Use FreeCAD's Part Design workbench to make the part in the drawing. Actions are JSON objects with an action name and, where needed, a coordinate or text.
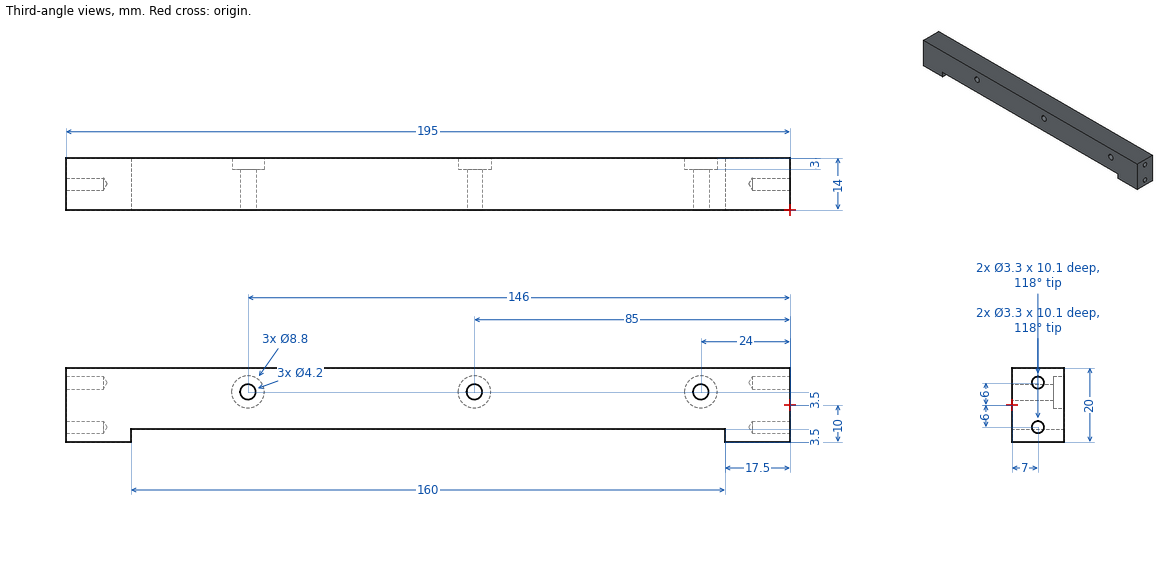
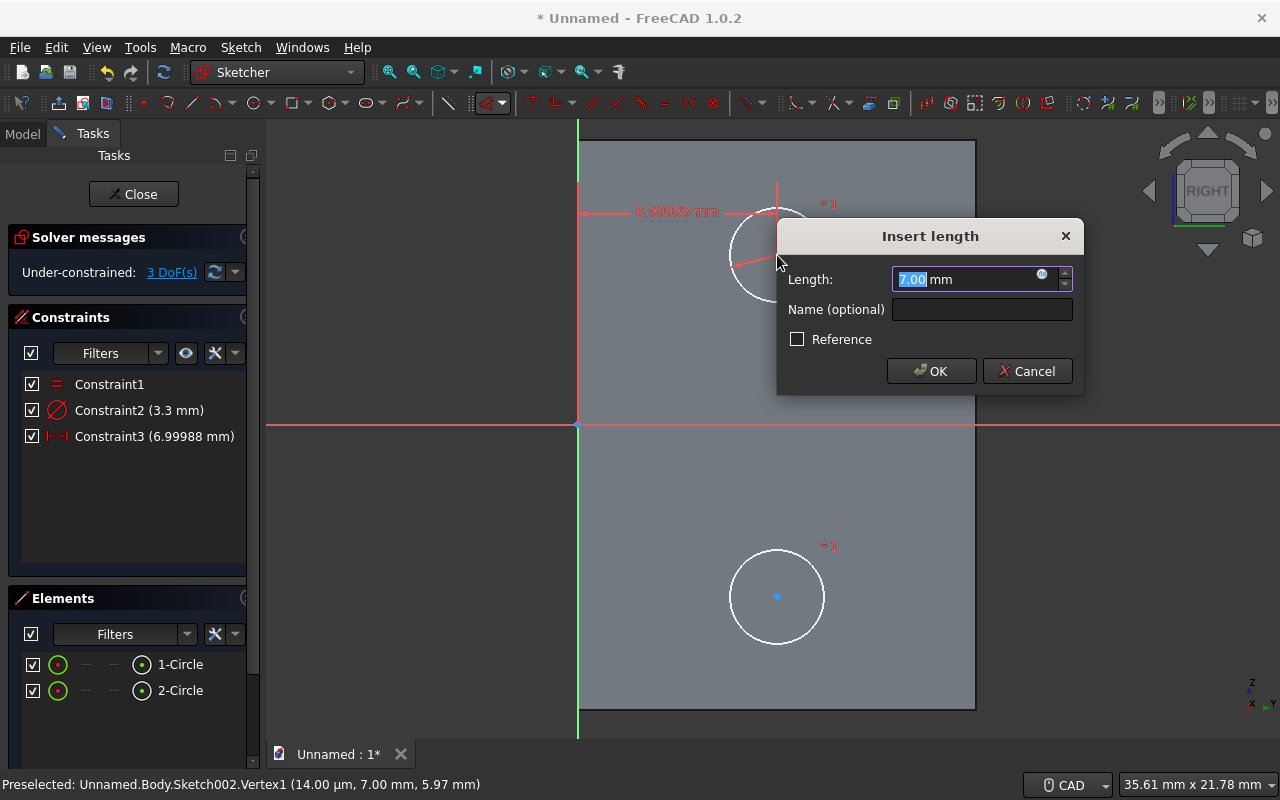
{"action": "type", "text": "7"}
{"action": "key", "text": "Return"}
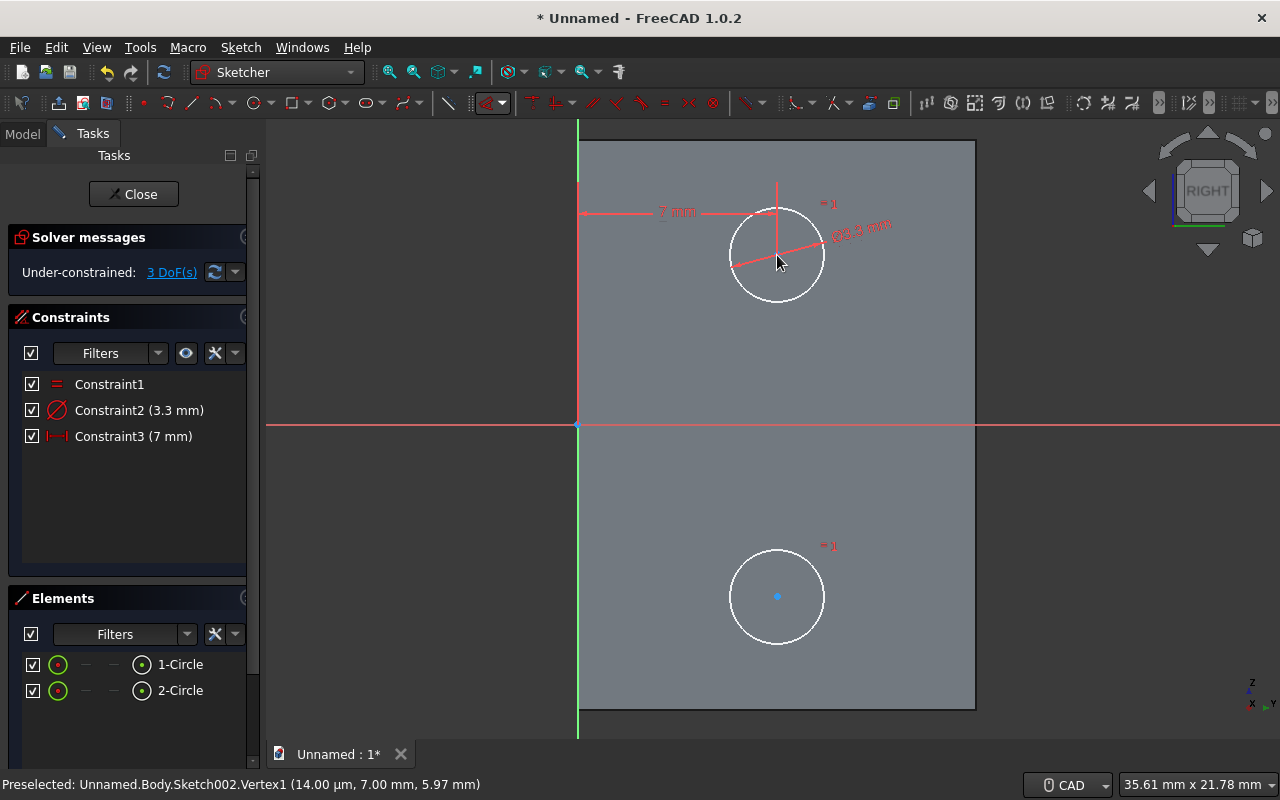
{"action": "left_click", "coordinate": [777, 255]}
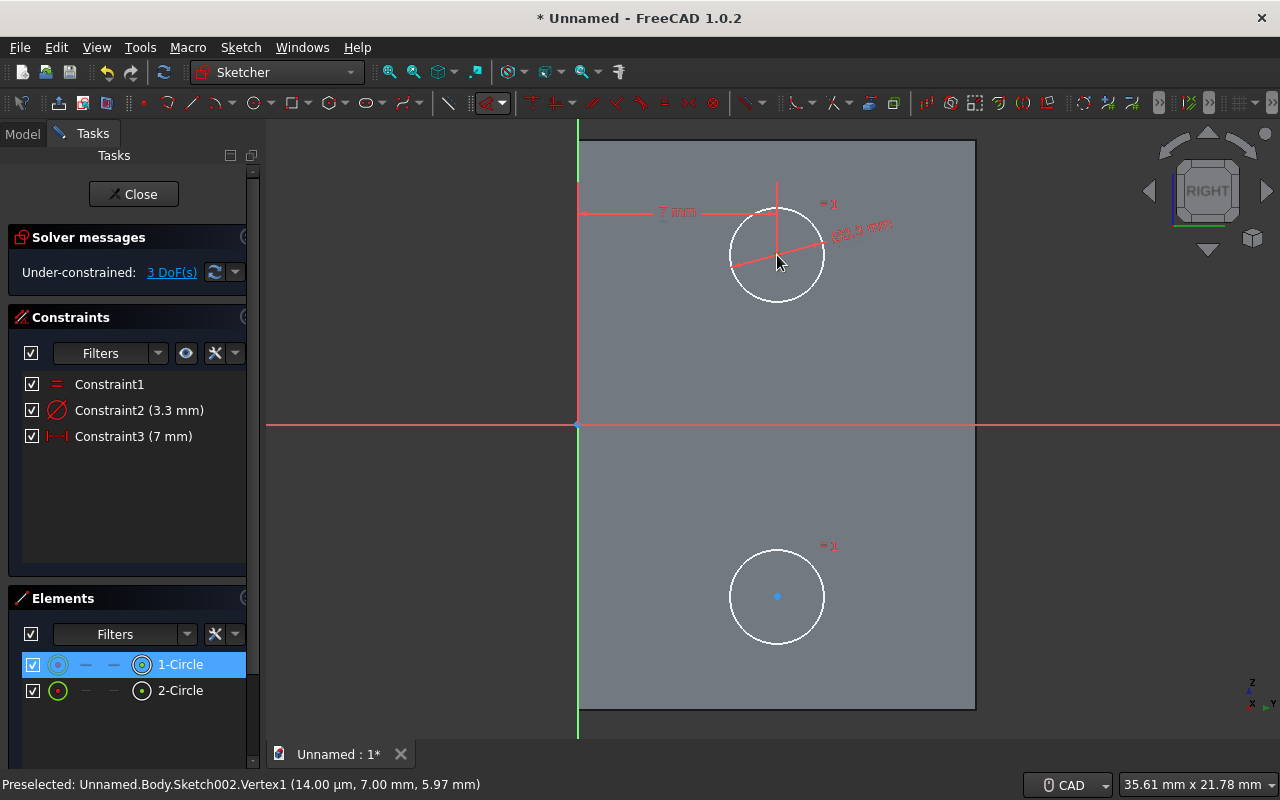
{"action": "key", "text": "i"}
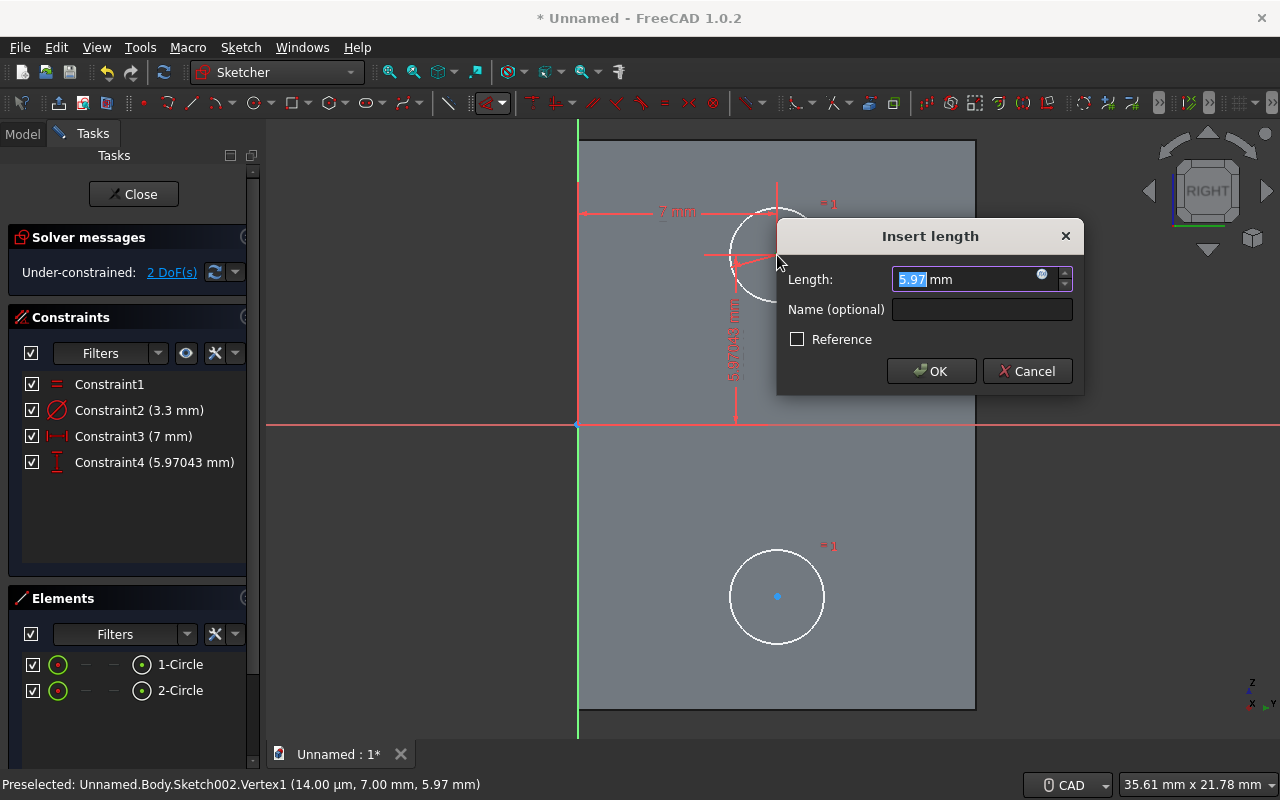
{"action": "type", "text": "6"}
{"action": "key", "text": "Return"}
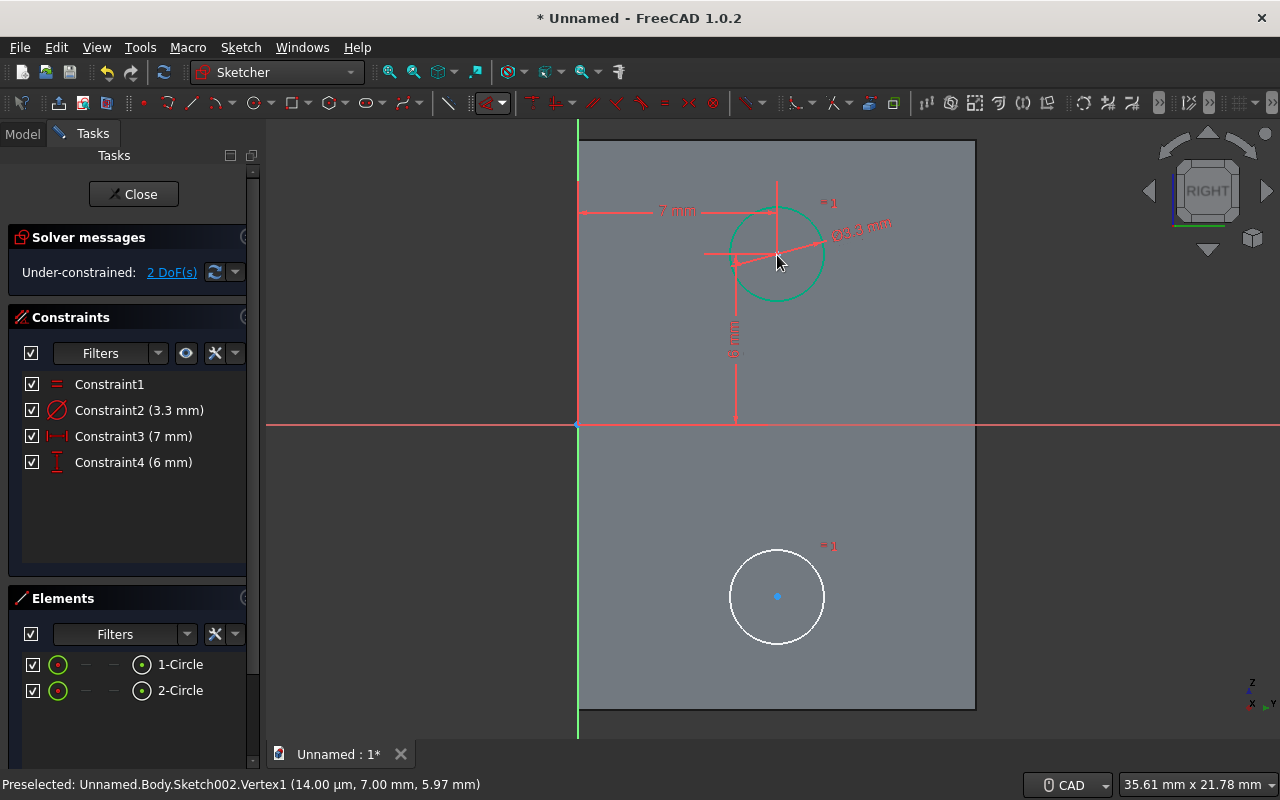
{"action": "left_click", "coordinate": [777, 597]}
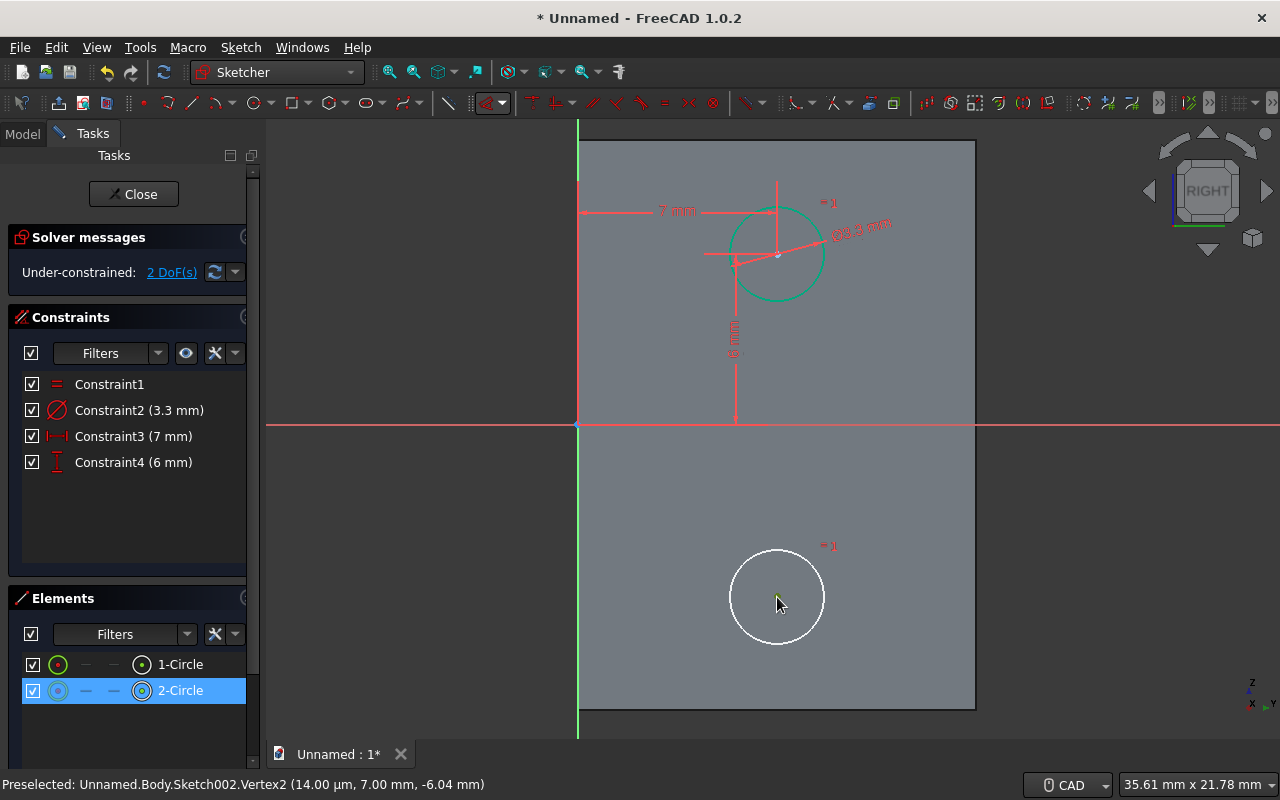
{"action": "key", "text": "l"}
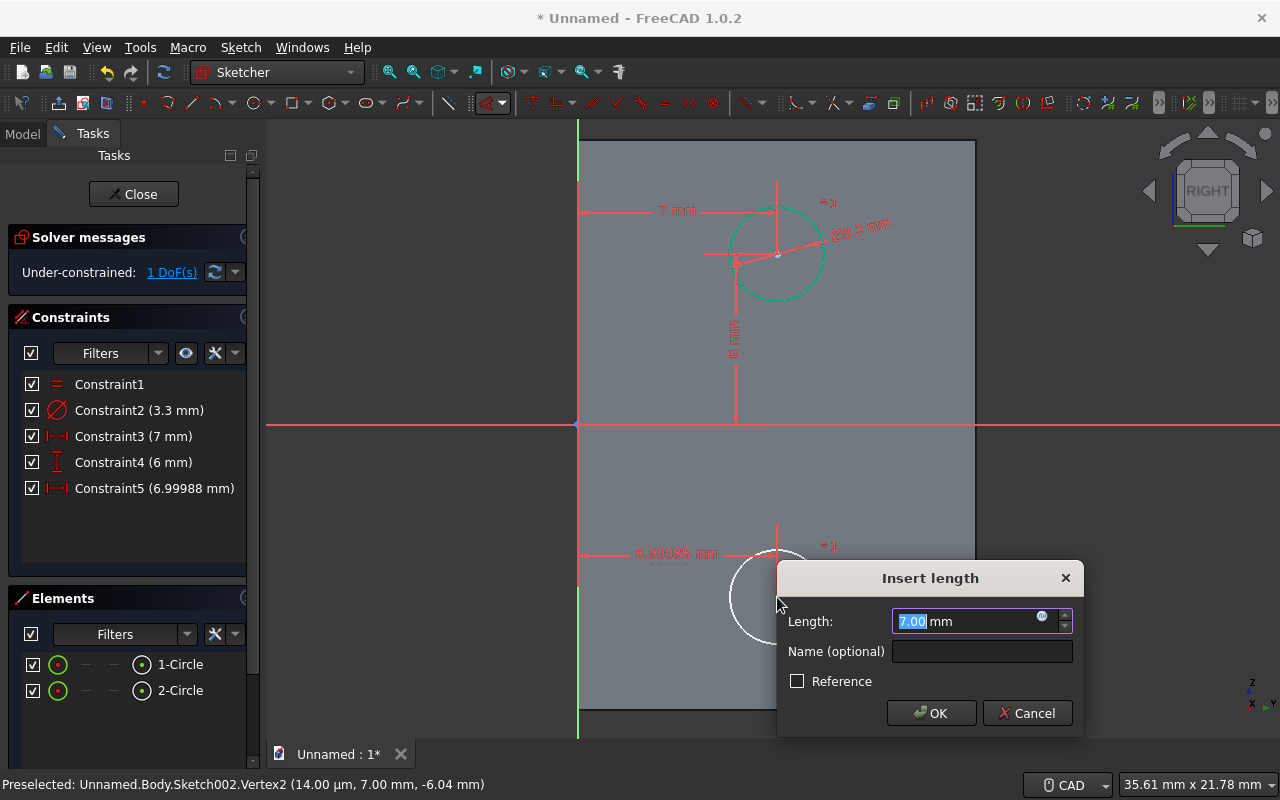
{"action": "type", "text": "7"}
{"action": "key", "text": "Return"}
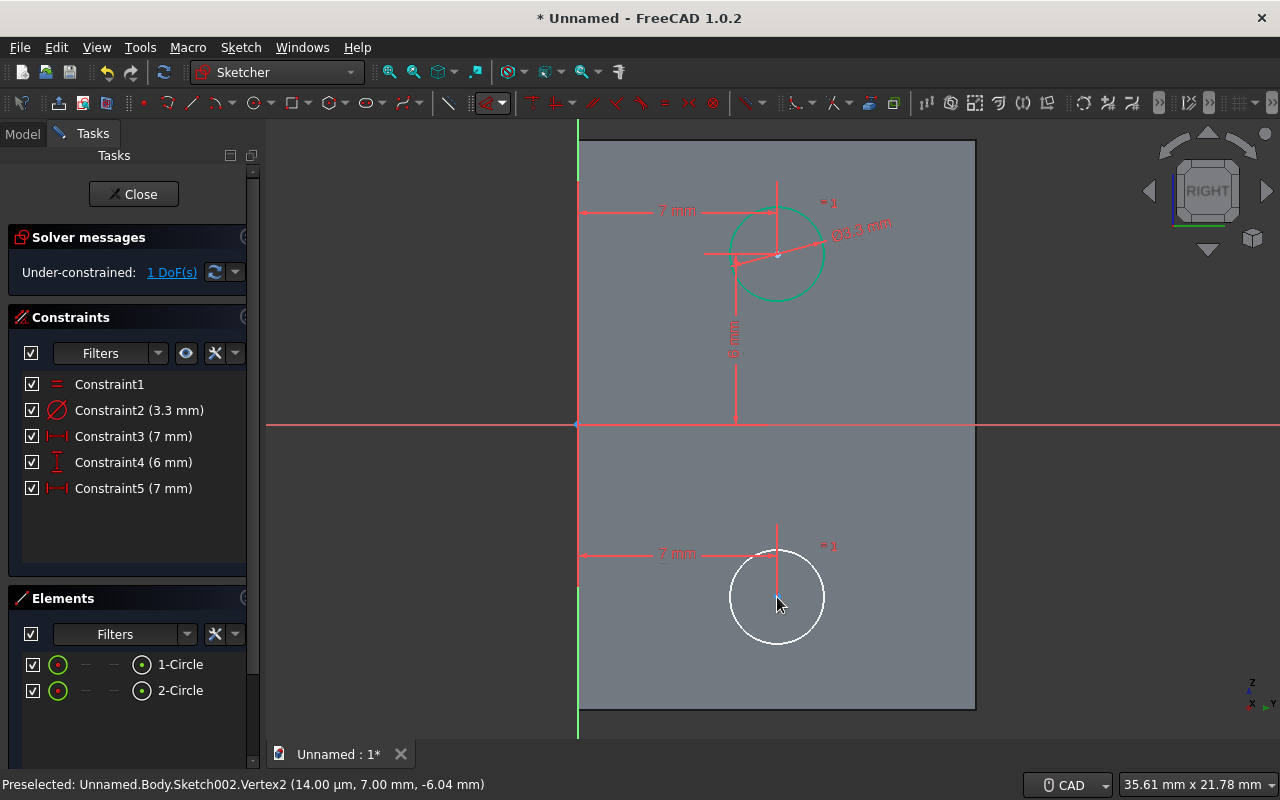
{"action": "left_click", "coordinate": [777, 597]}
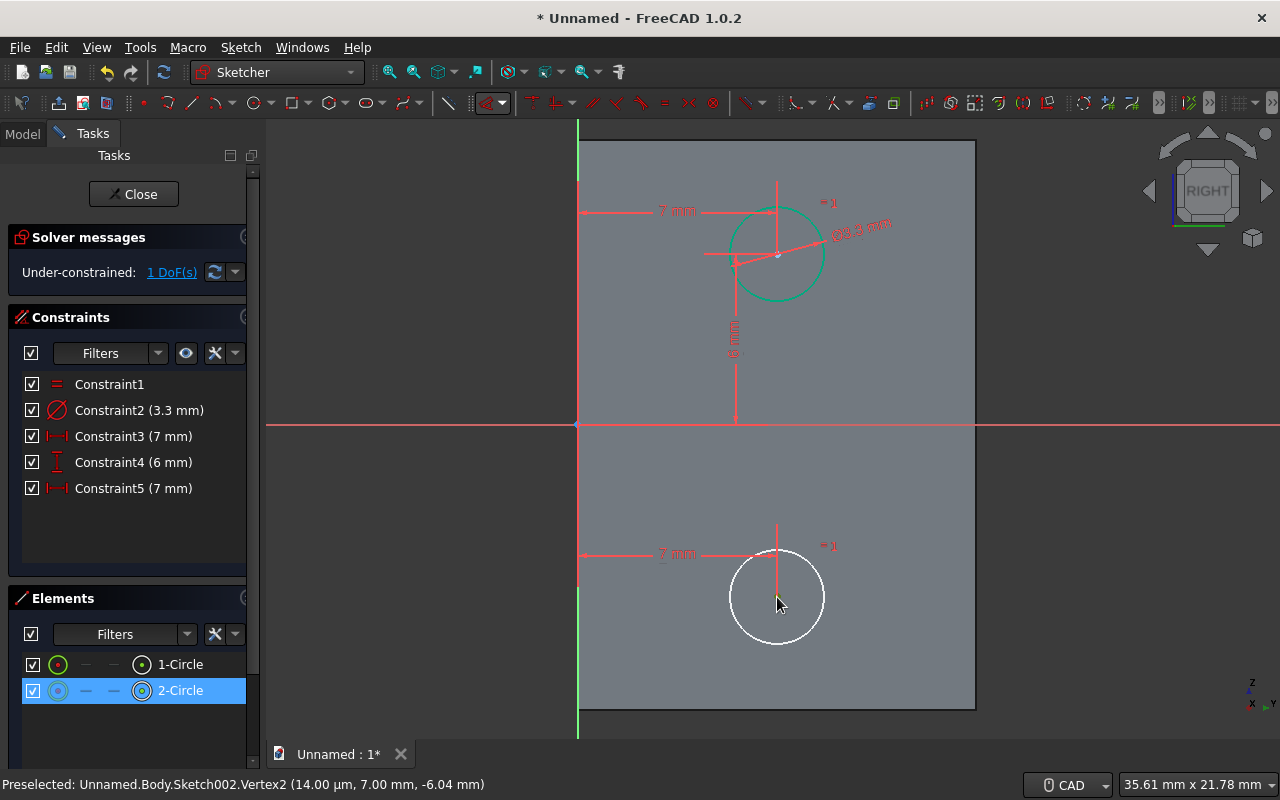
{"action": "left_click", "coordinate": [504, 104]}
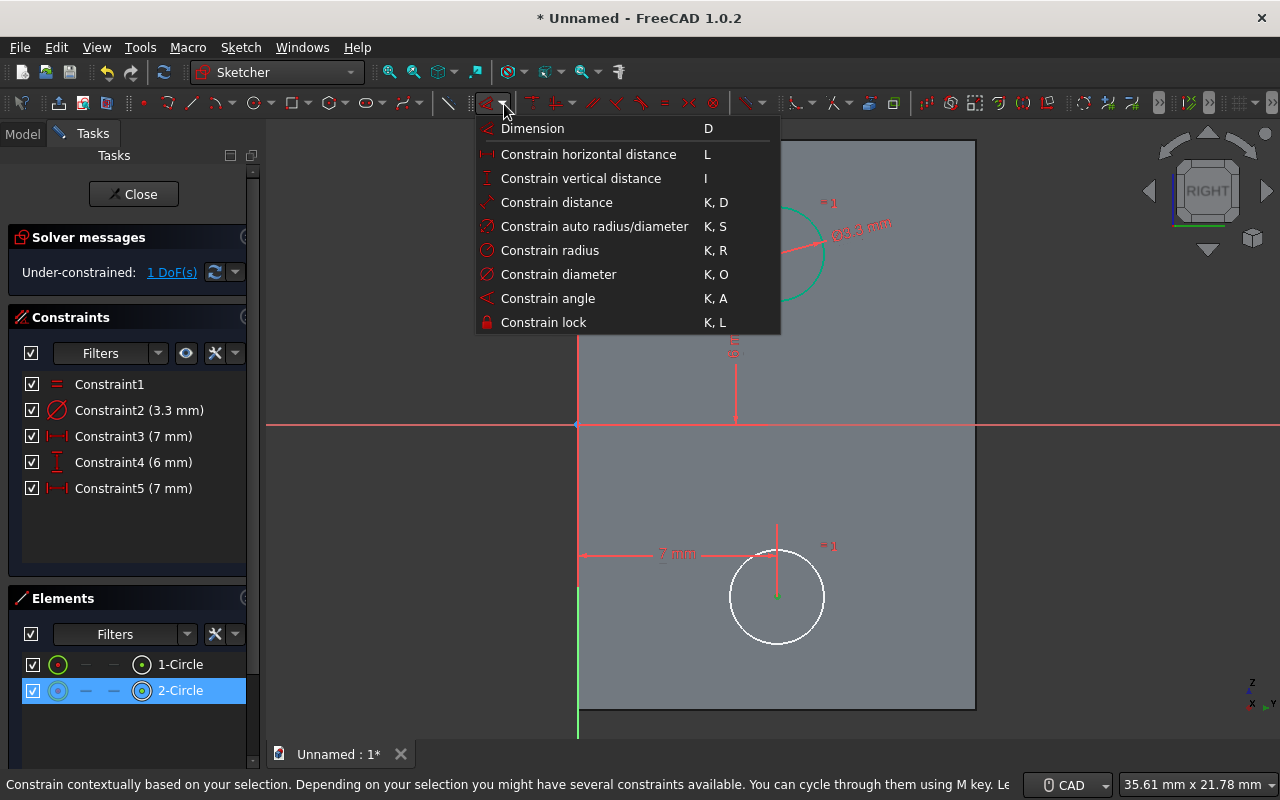
{"action": "left_click", "coordinate": [628, 178]}